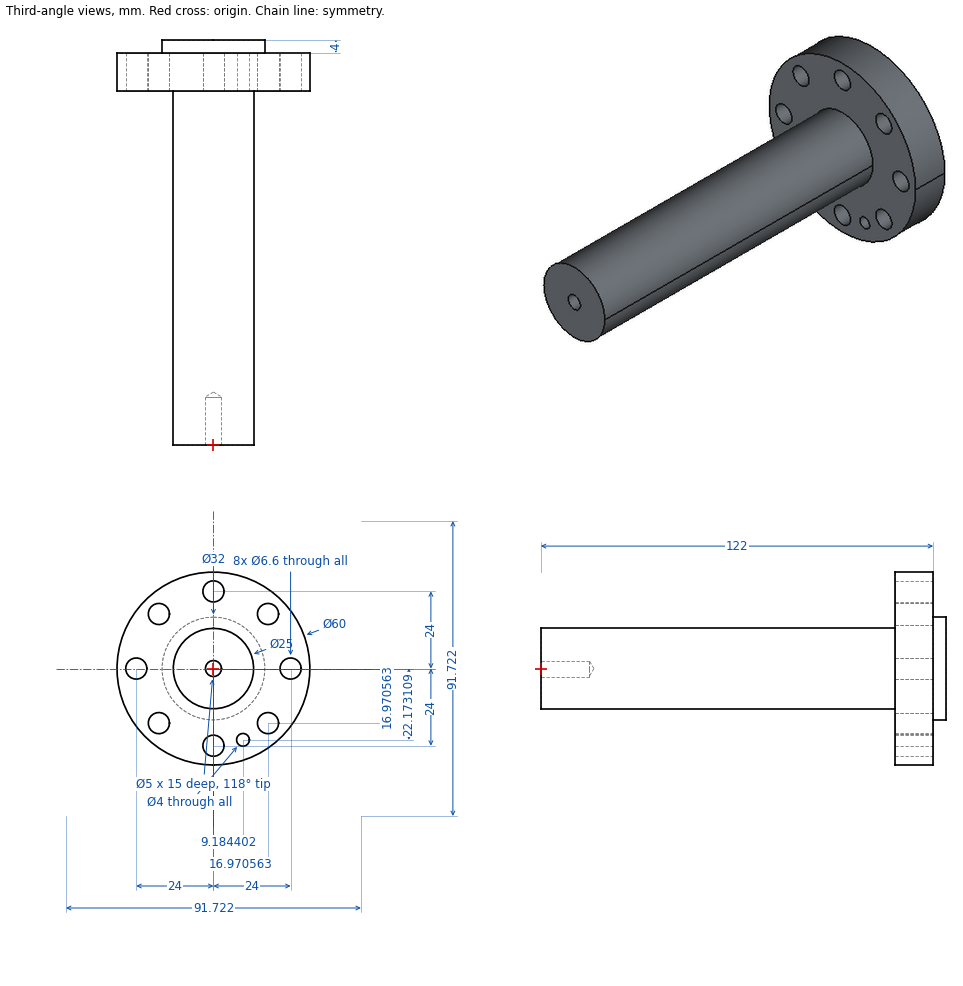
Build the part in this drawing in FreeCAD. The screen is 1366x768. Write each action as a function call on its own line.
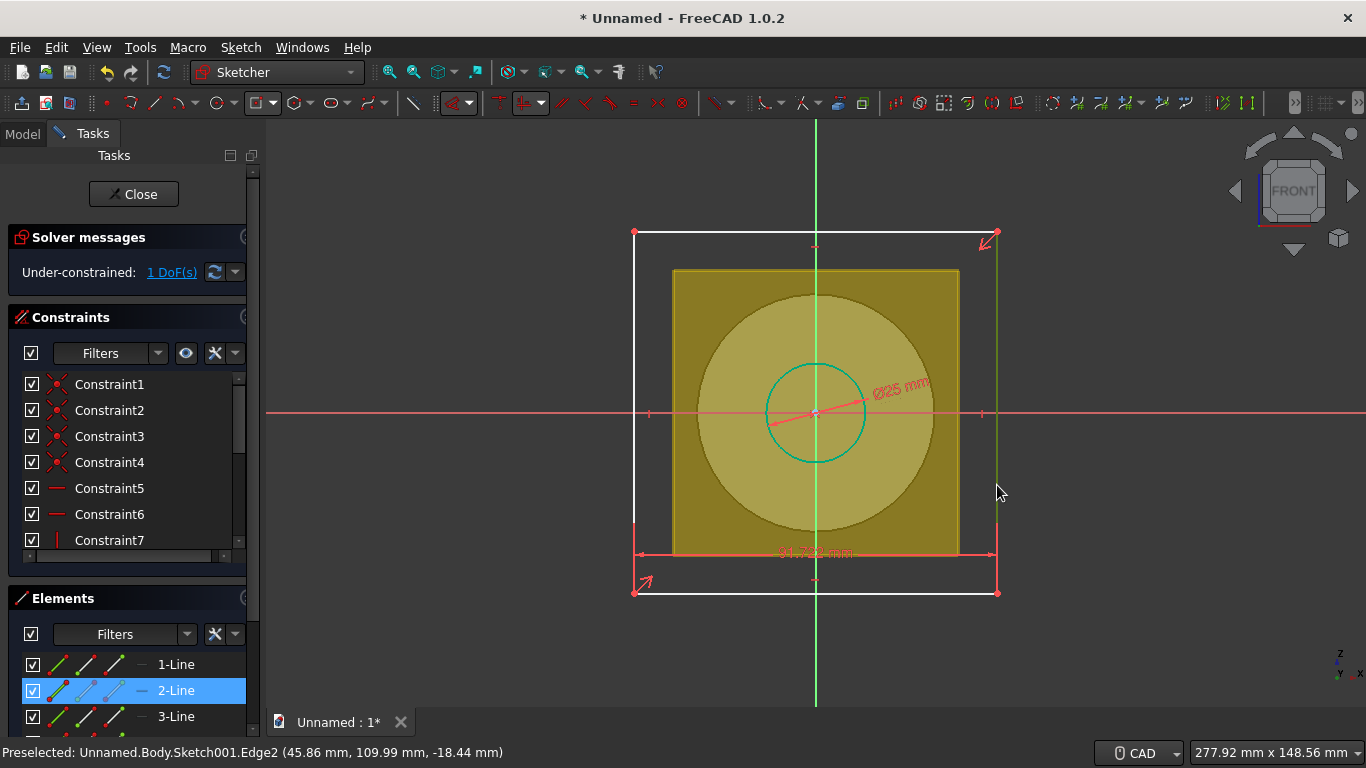
click(472, 104)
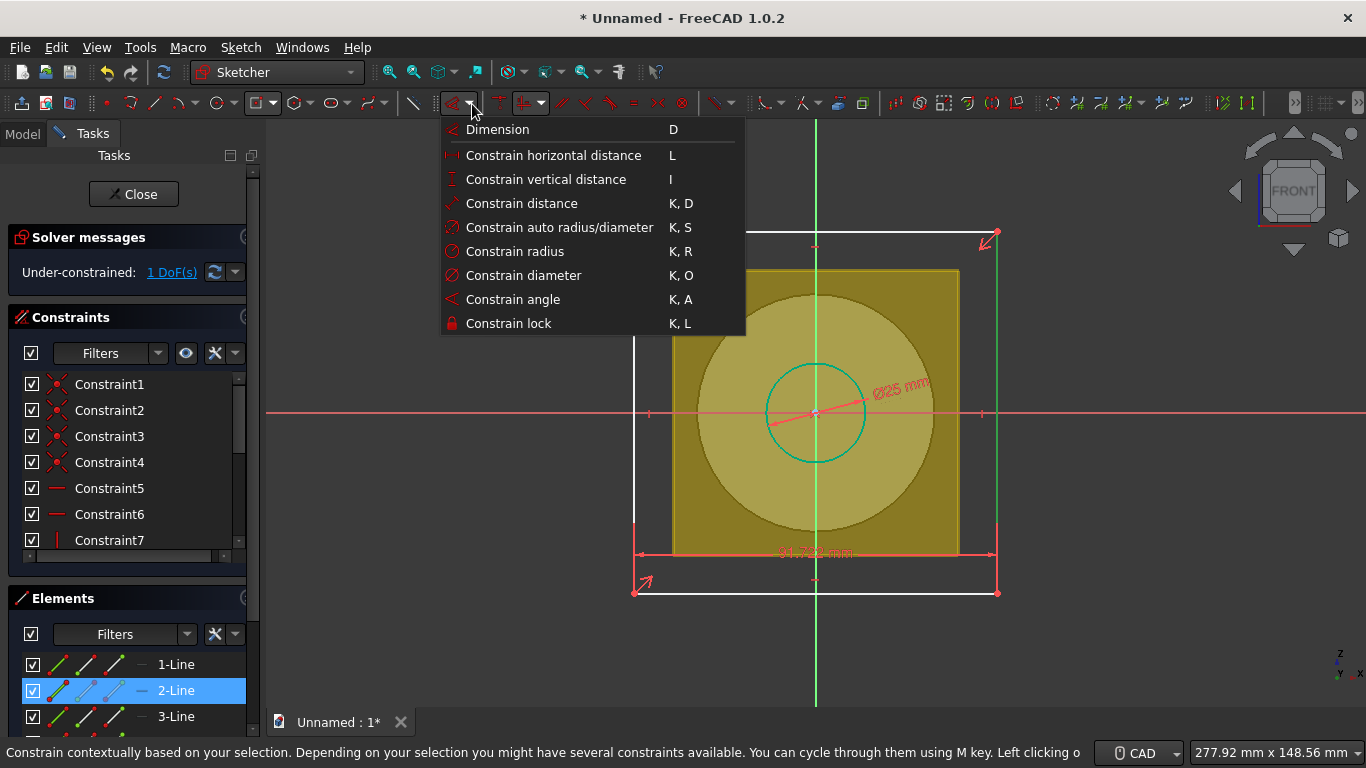
click(593, 179)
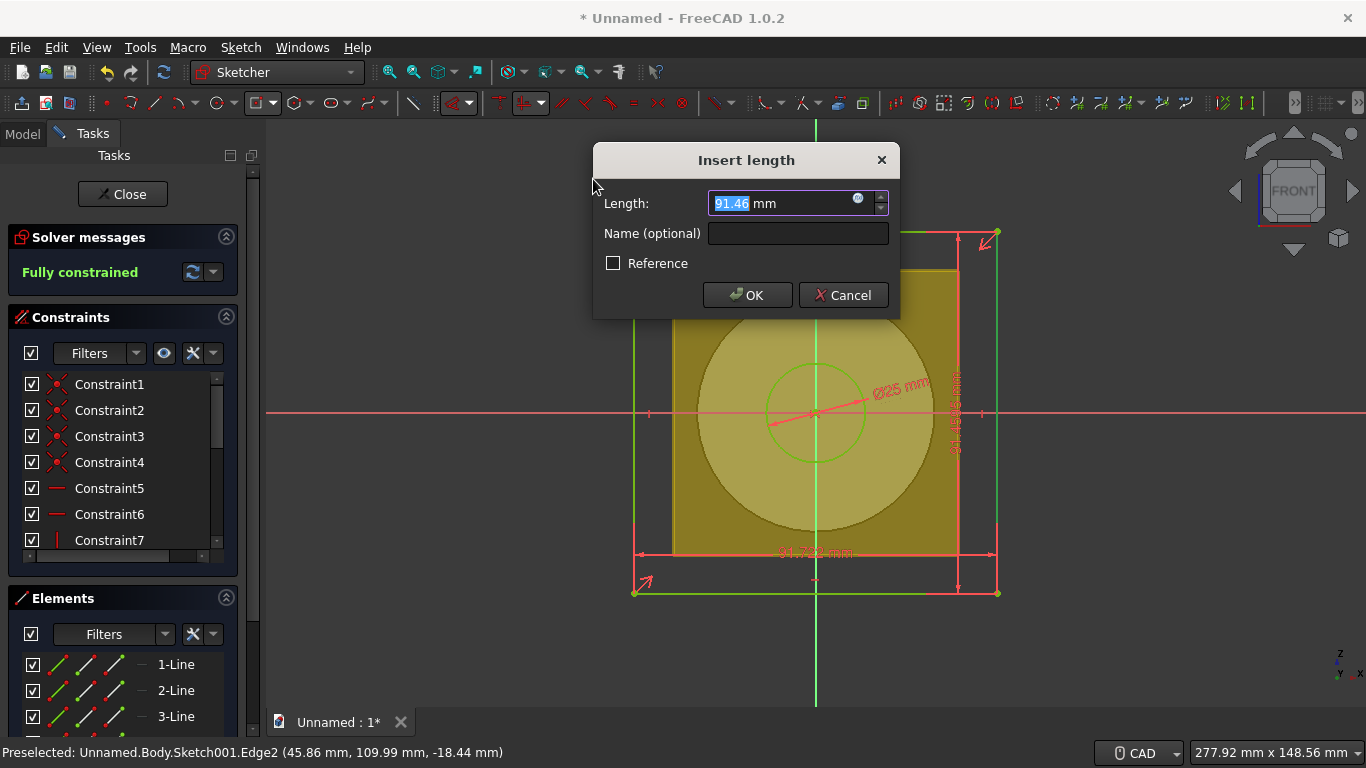
text(91.722)
key(Return)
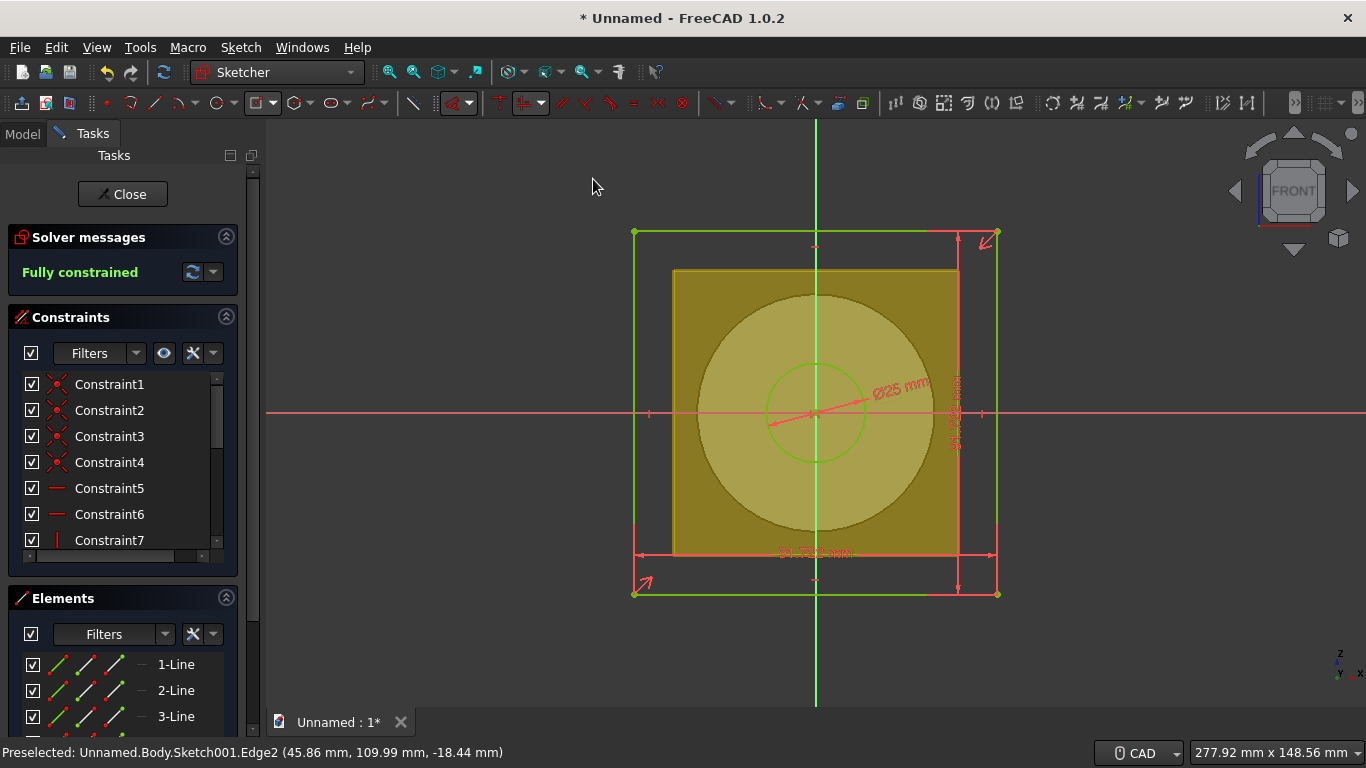
click(123, 194)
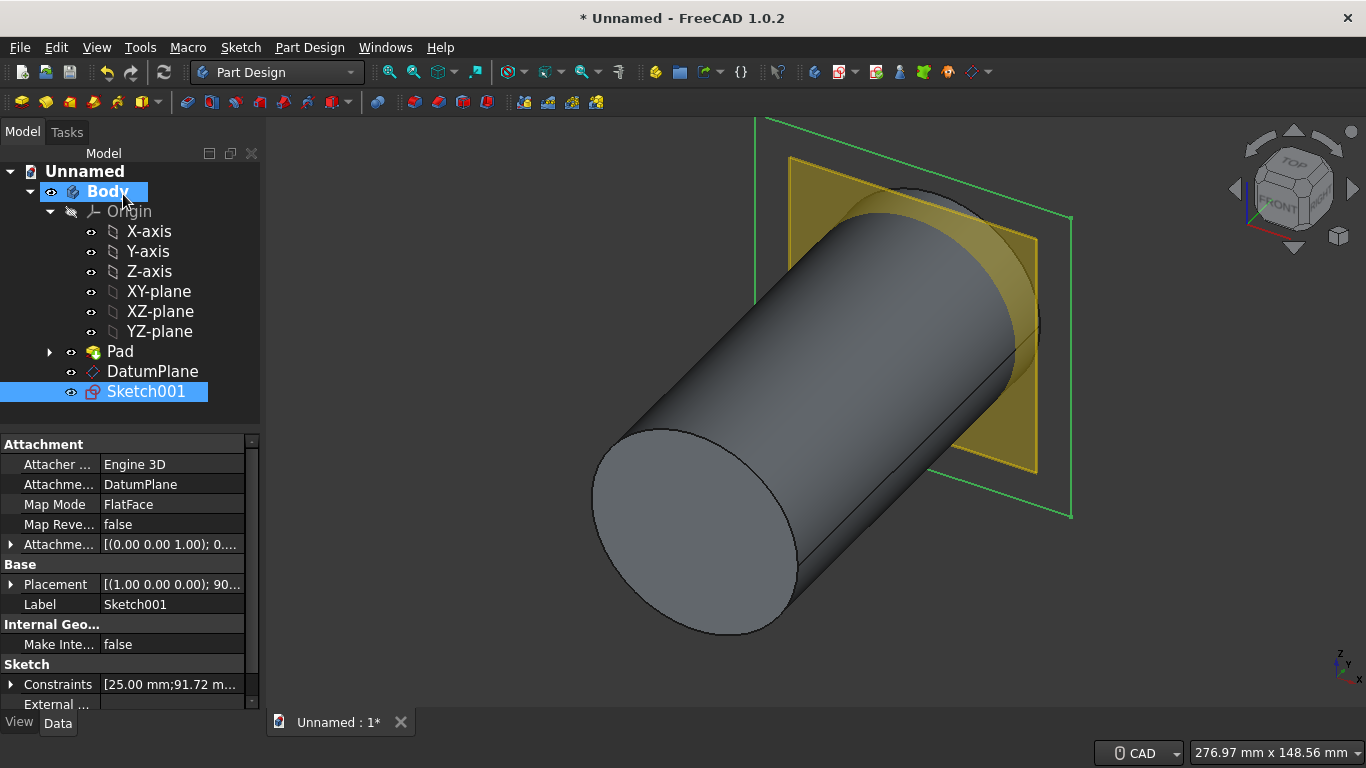
click(188, 102)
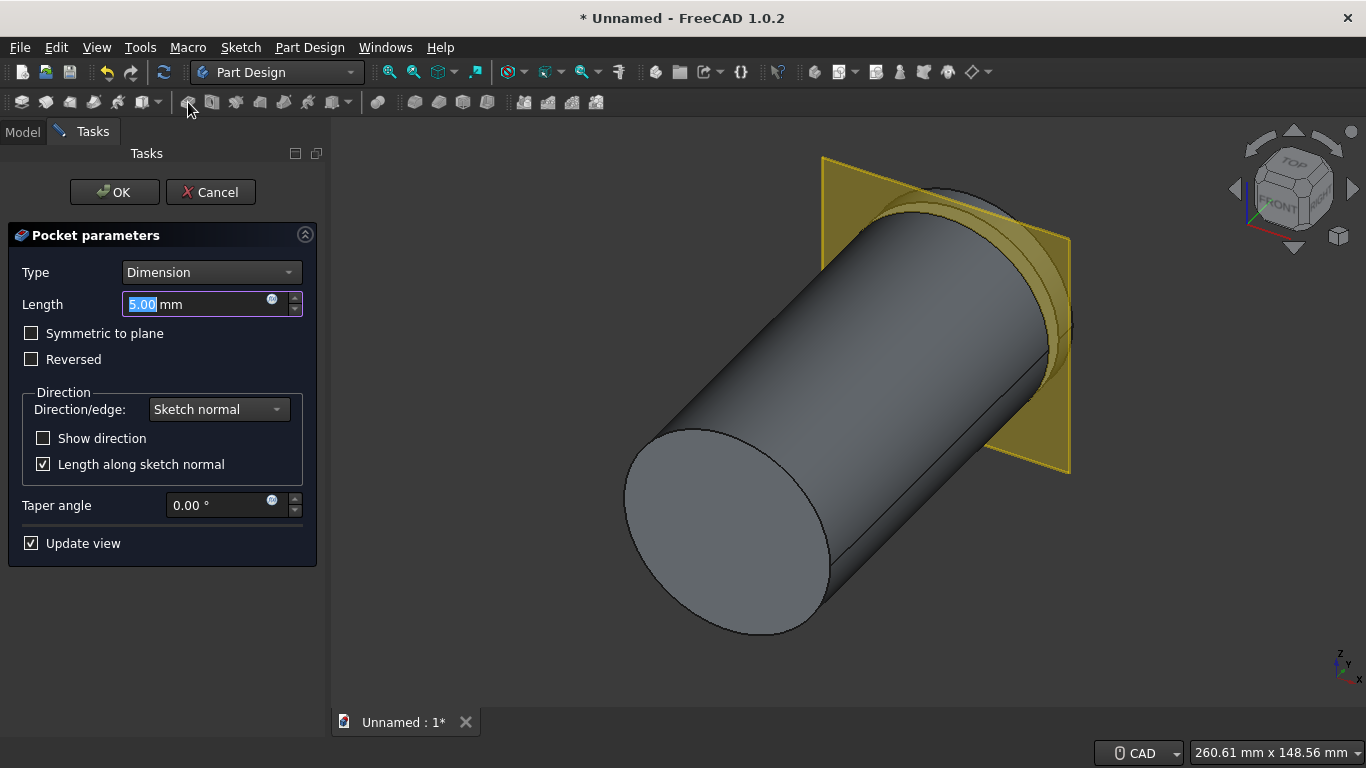
click(212, 272)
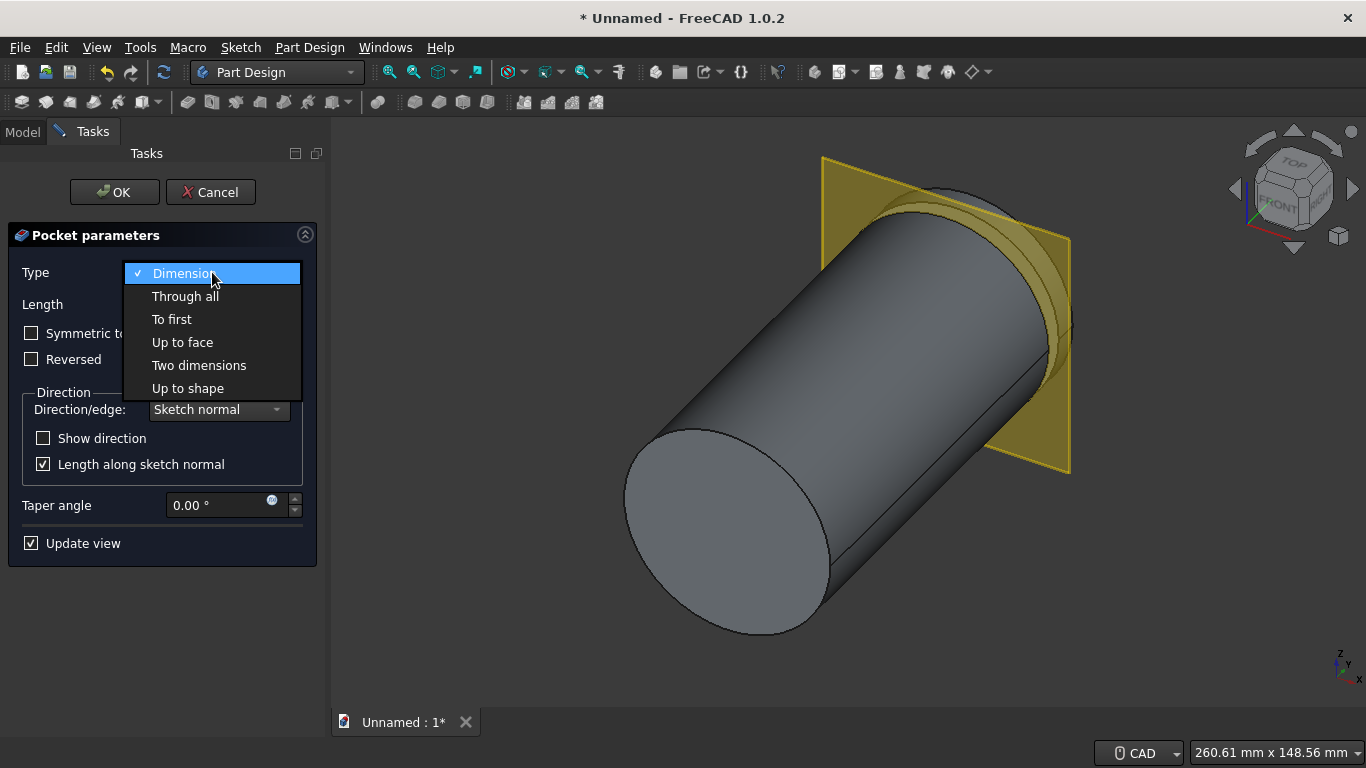
click(212, 296)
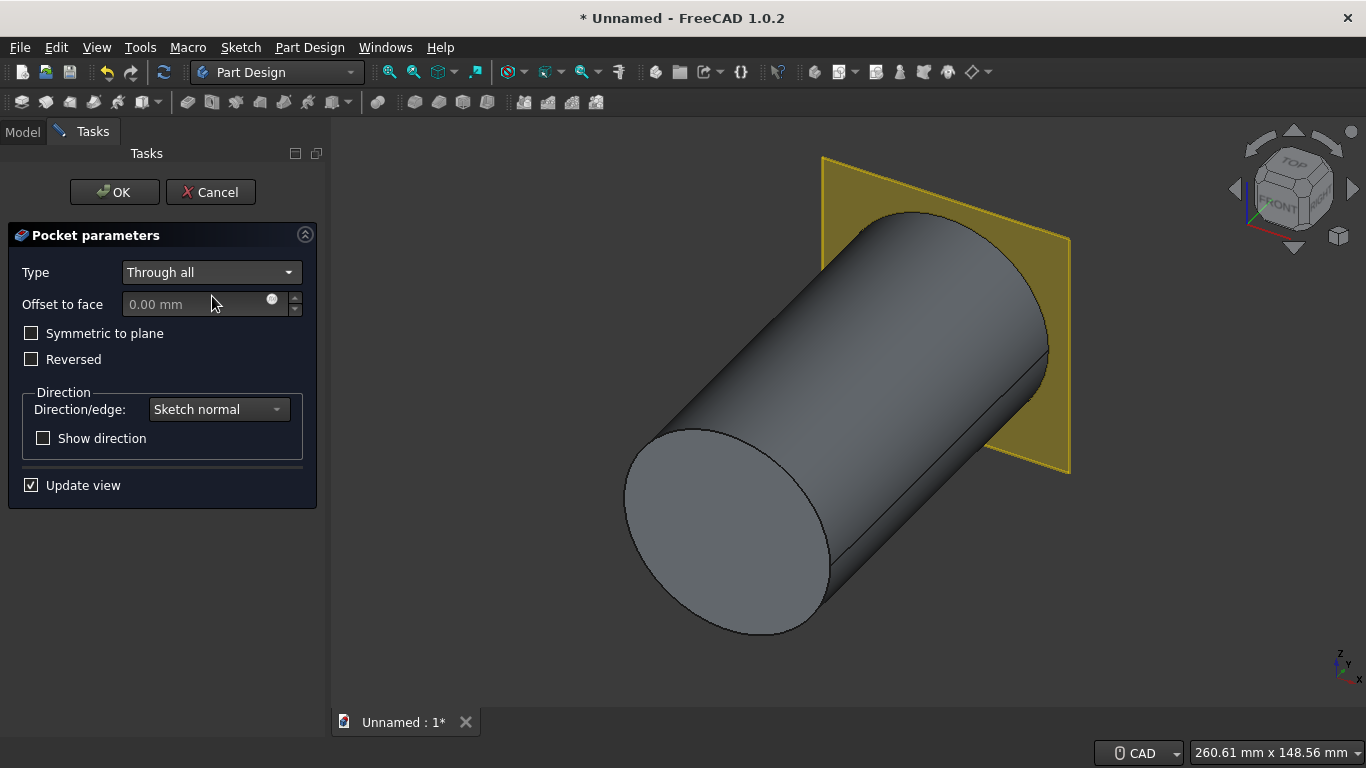
click(30, 359)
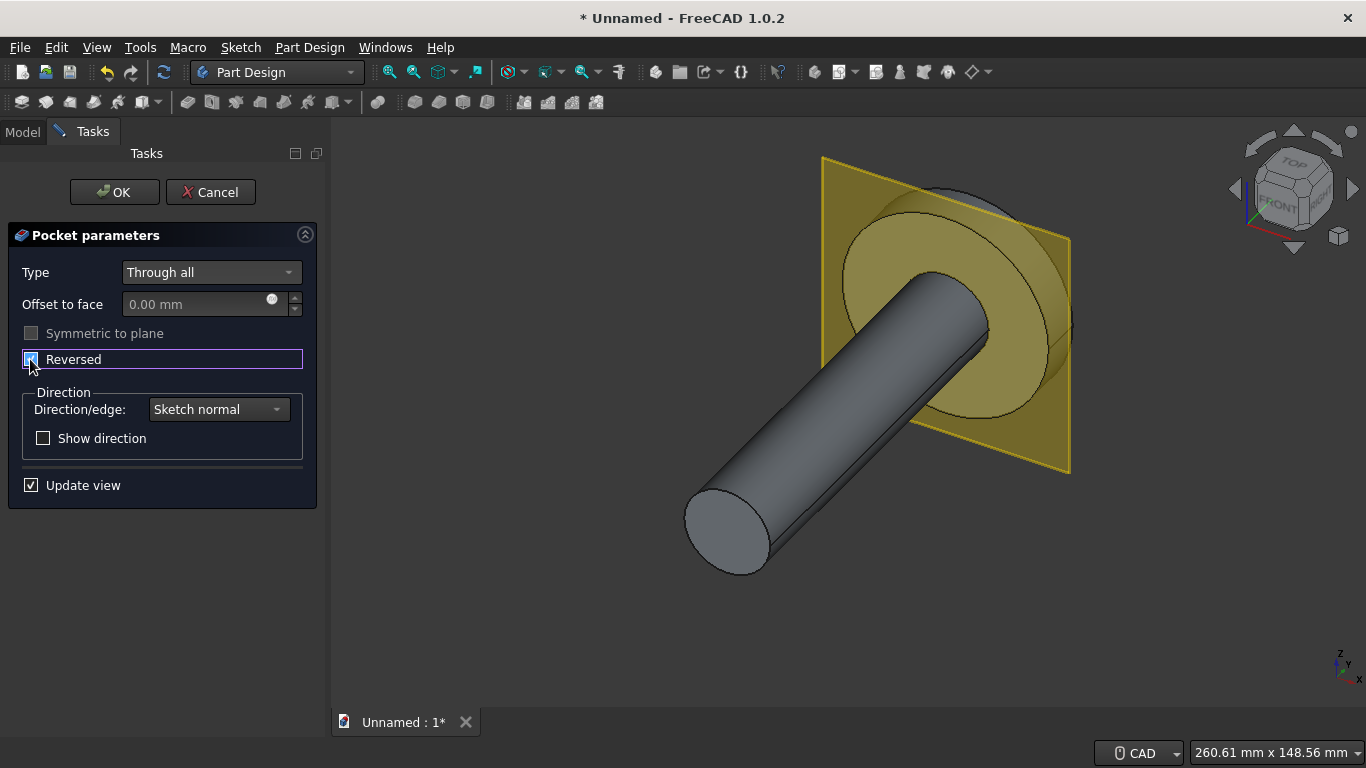
click(115, 192)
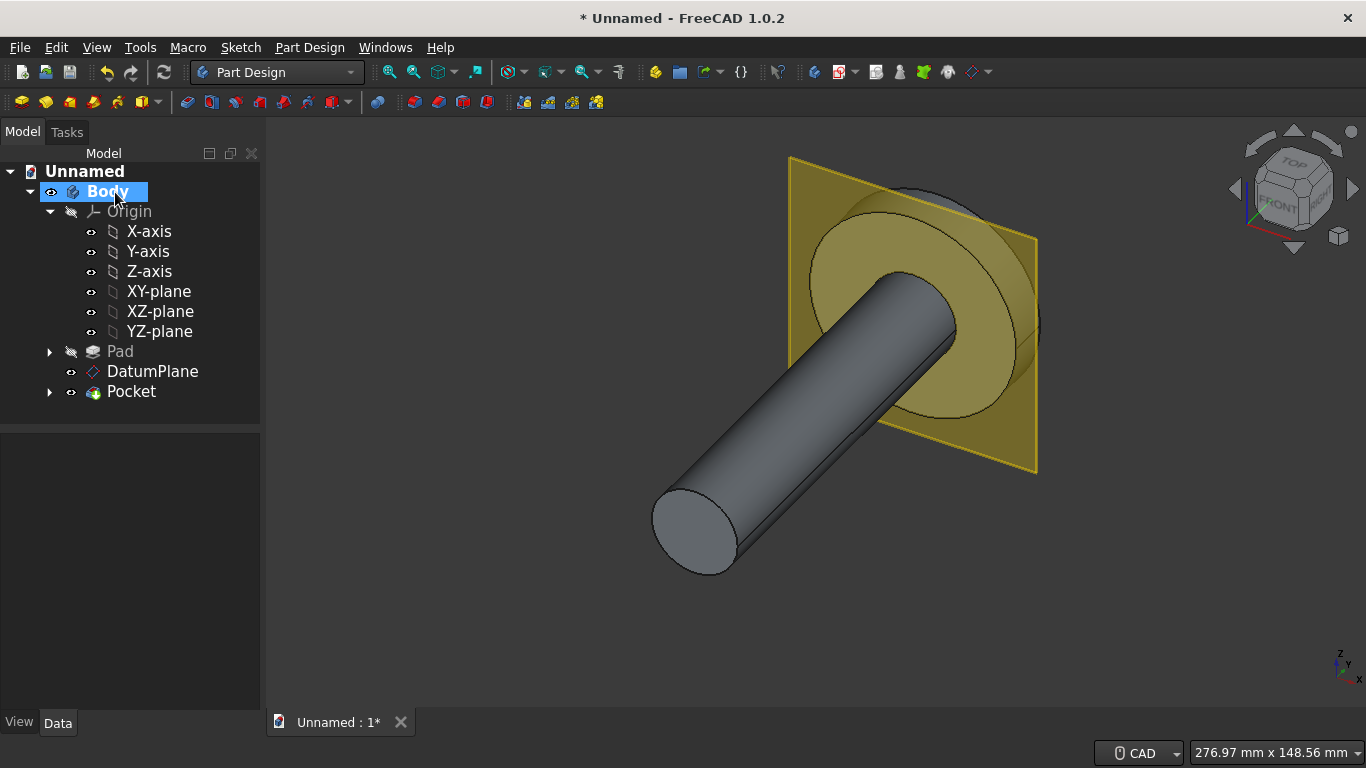
click(116, 372)
key(space)